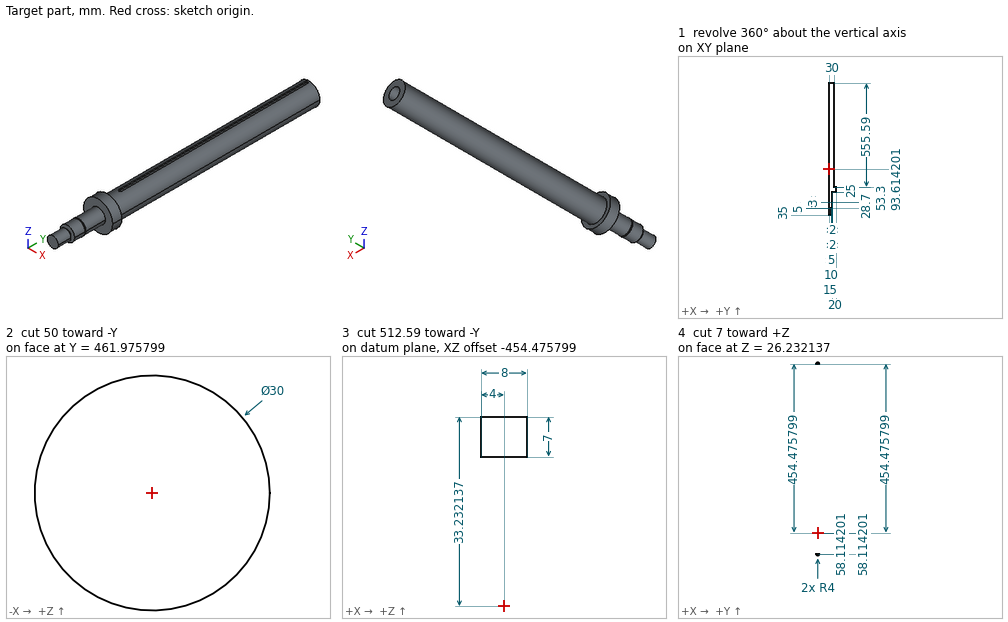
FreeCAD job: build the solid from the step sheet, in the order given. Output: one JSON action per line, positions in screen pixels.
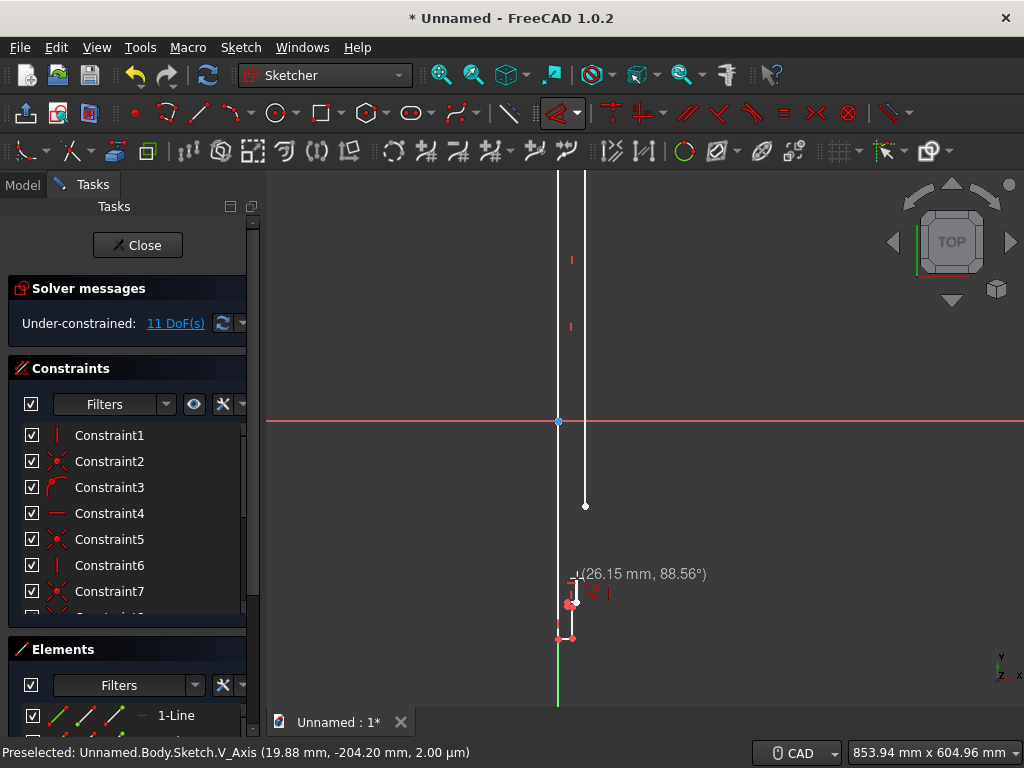
{"action": "left_click", "coordinate": [576, 577]}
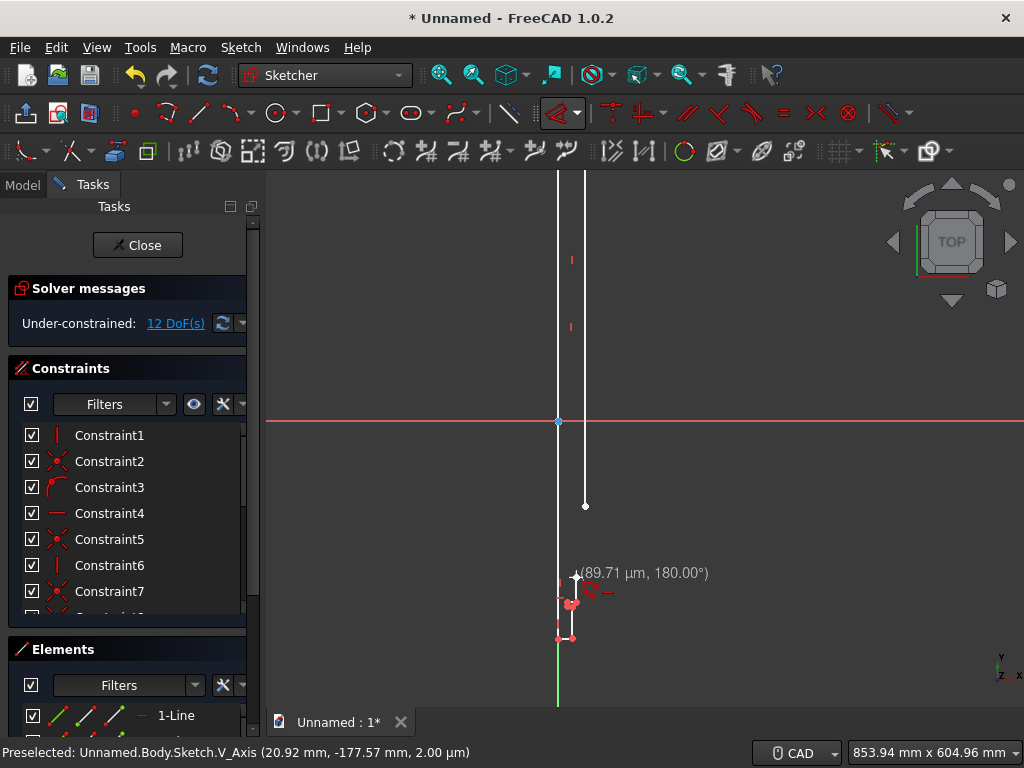
{"action": "scroll", "coordinate": [574, 577], "scroll_direction": "up", "scroll_amount": 11}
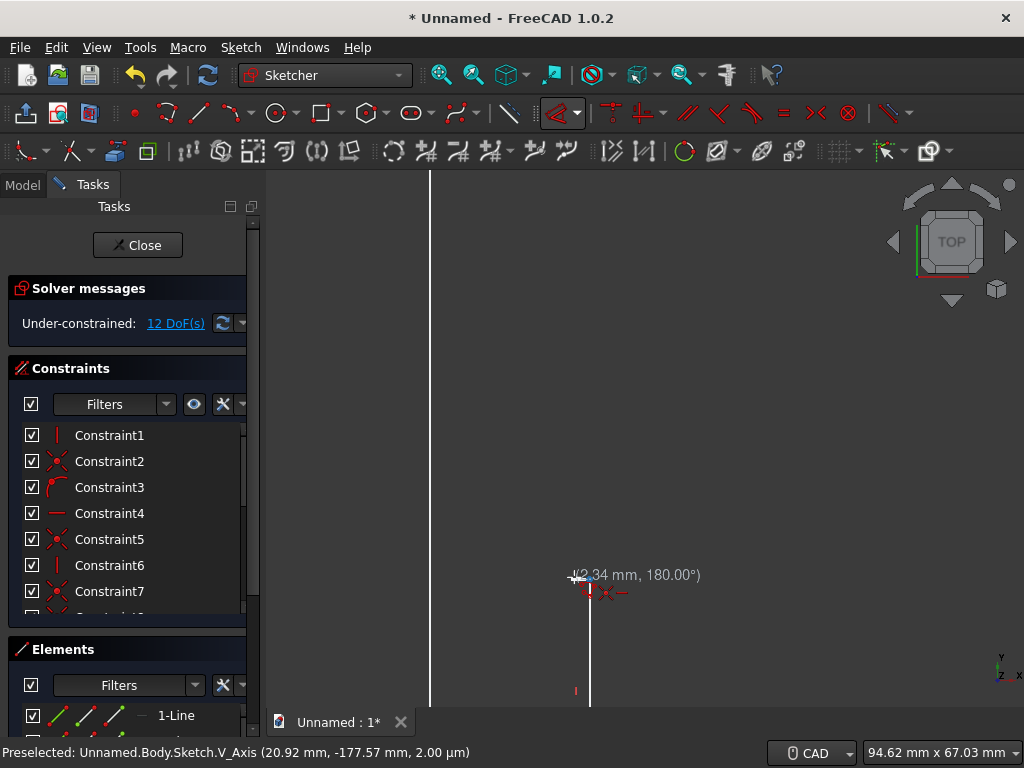
{"action": "left_click", "coordinate": [574, 571]}
{"action": "left_click", "coordinate": [574, 544]}
{"action": "left_click", "coordinate": [590, 544]}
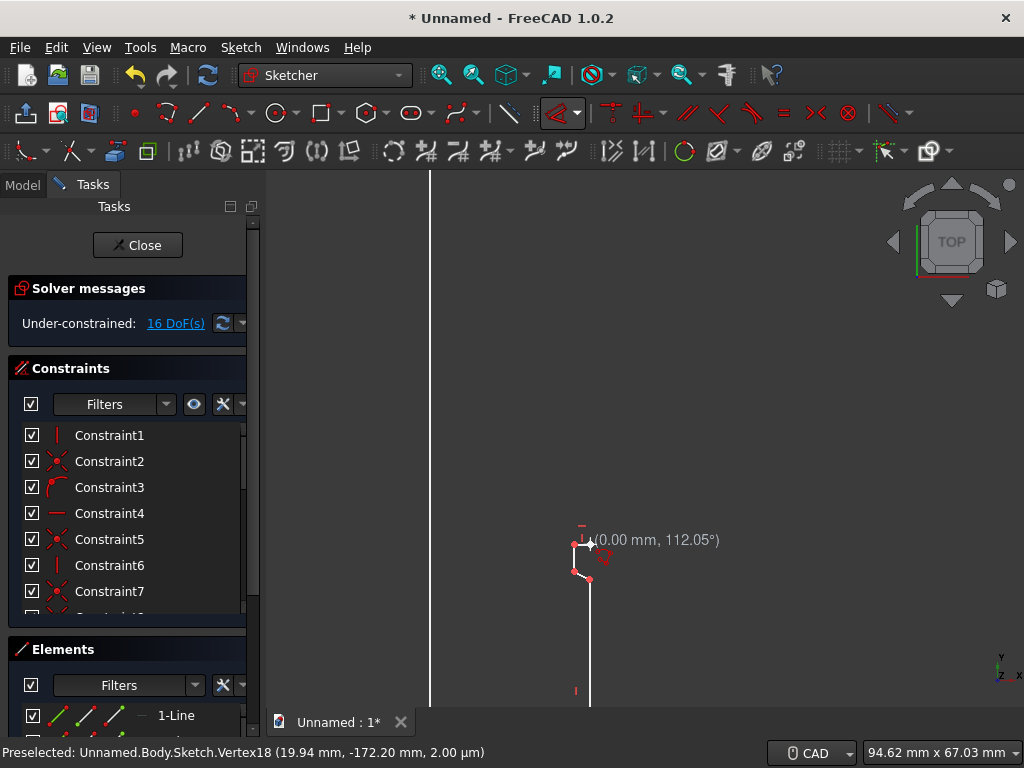
{"action": "scroll", "coordinate": [576, 577], "scroll_direction": "down", "scroll_amount": 14}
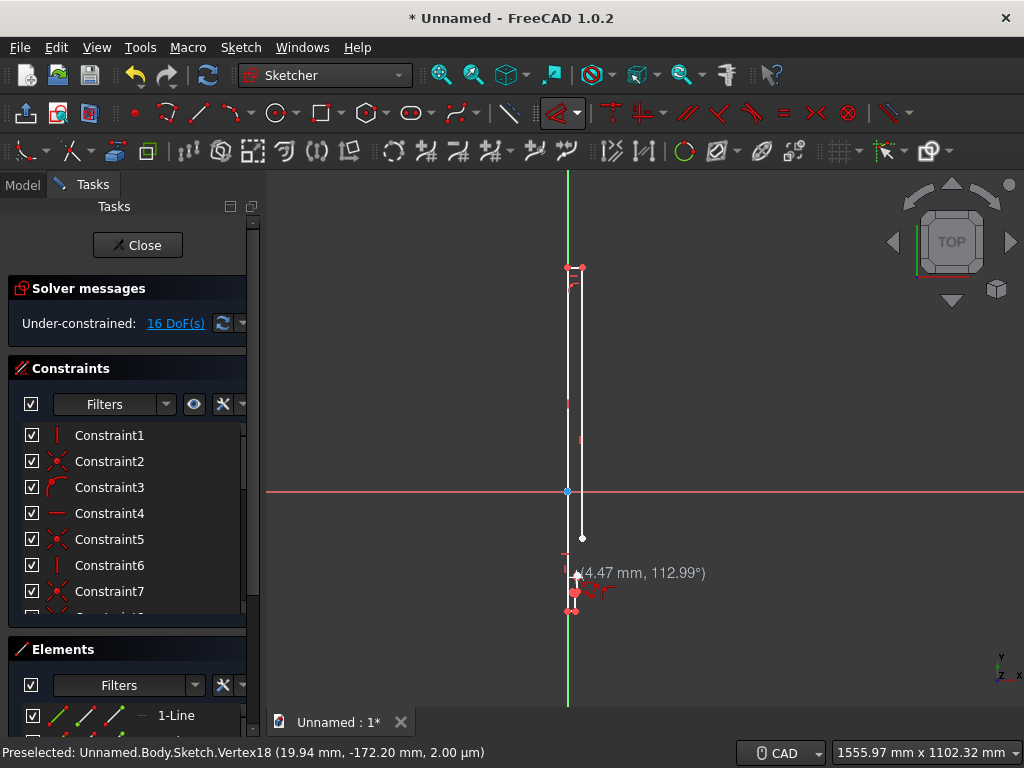
{"action": "scroll", "coordinate": [577, 550], "scroll_direction": "up", "scroll_amount": 3}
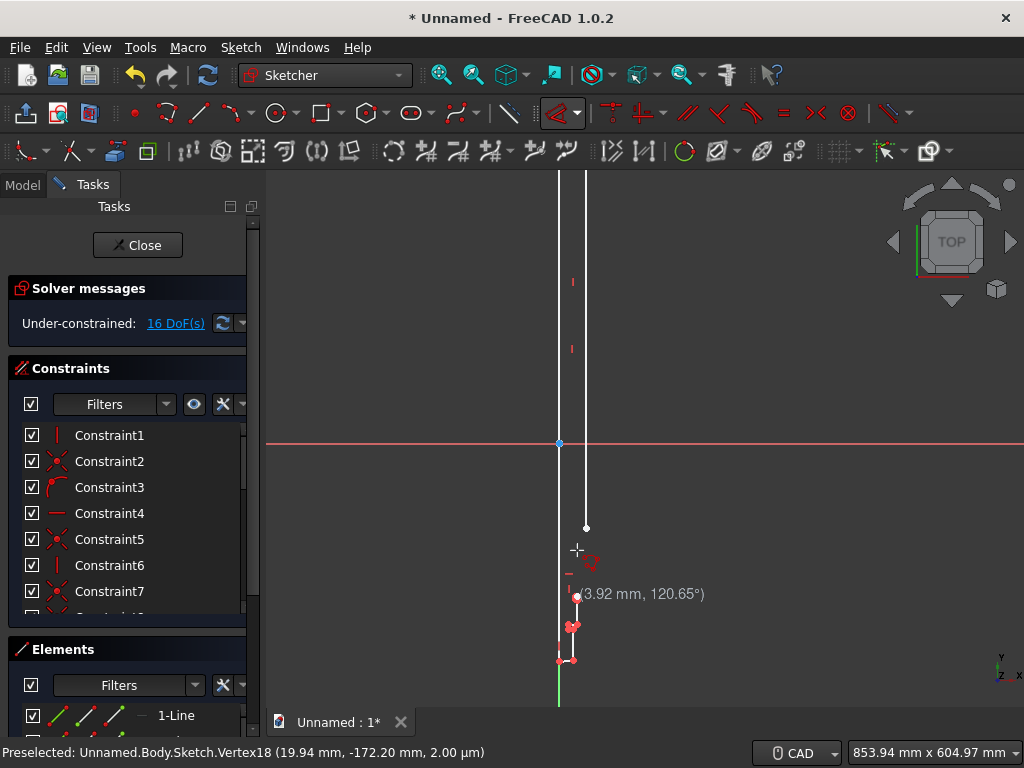
{"action": "left_click", "coordinate": [577, 549]}
{"action": "left_click", "coordinate": [595, 549]}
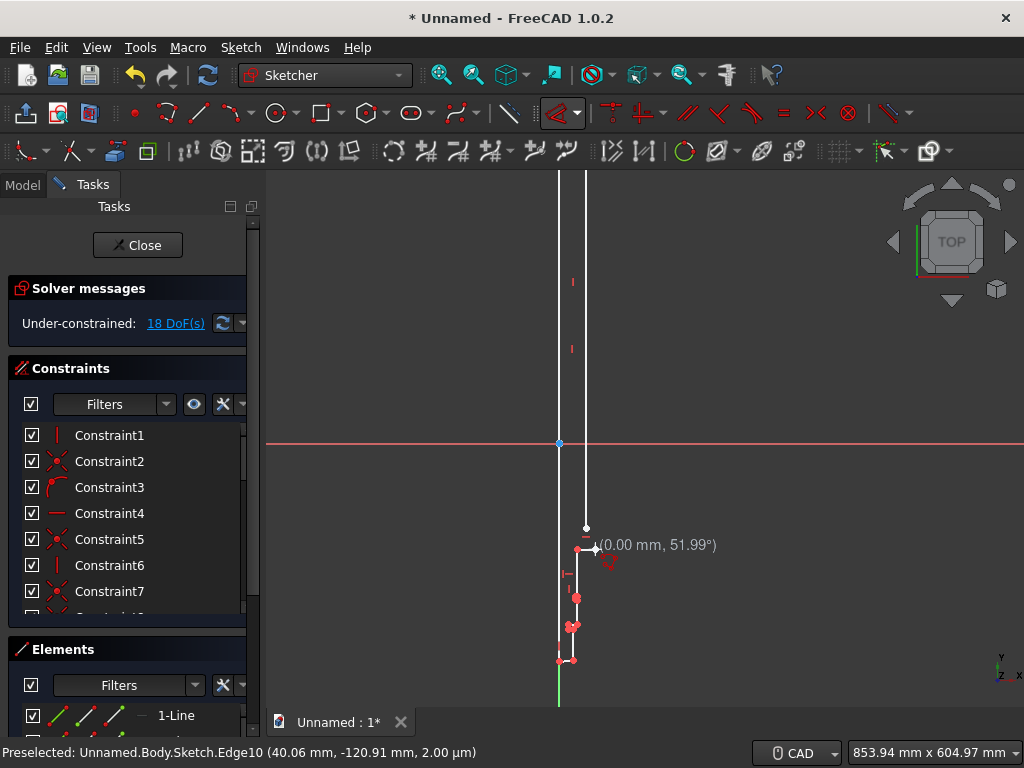
{"action": "scroll", "coordinate": [595, 527], "scroll_direction": "up", "scroll_amount": 3}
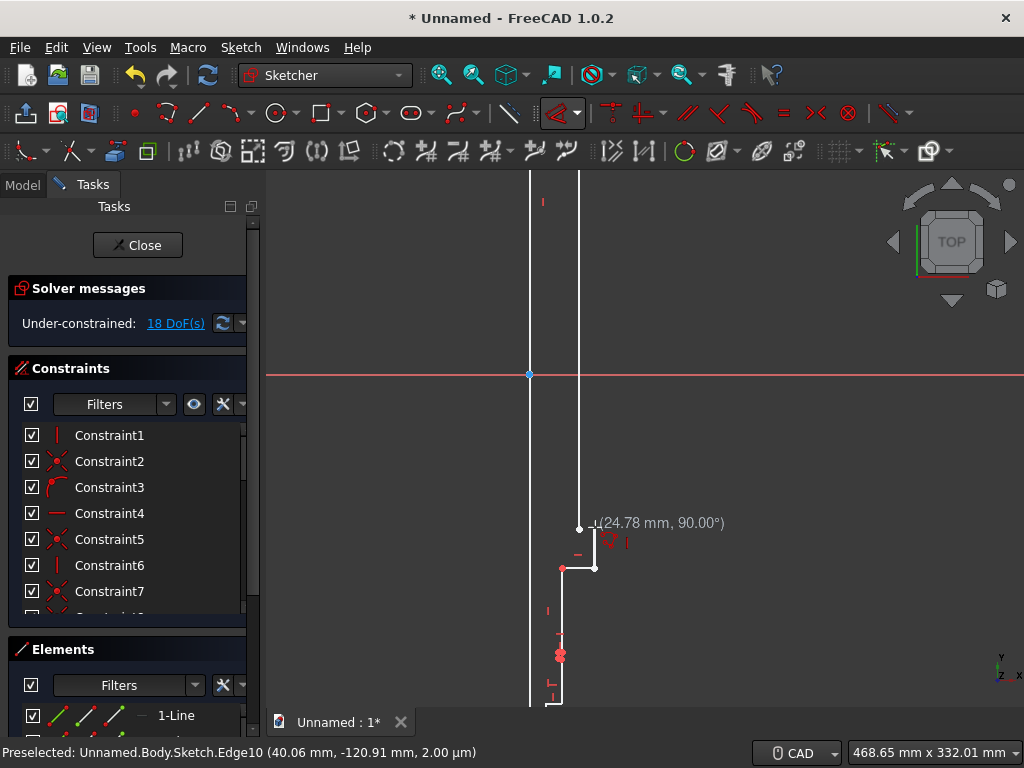
{"action": "left_click", "coordinate": [595, 526]}
{"action": "left_click", "coordinate": [579, 530]}
{"action": "key", "text": "Escape"}
{"action": "key", "text": "Escape"}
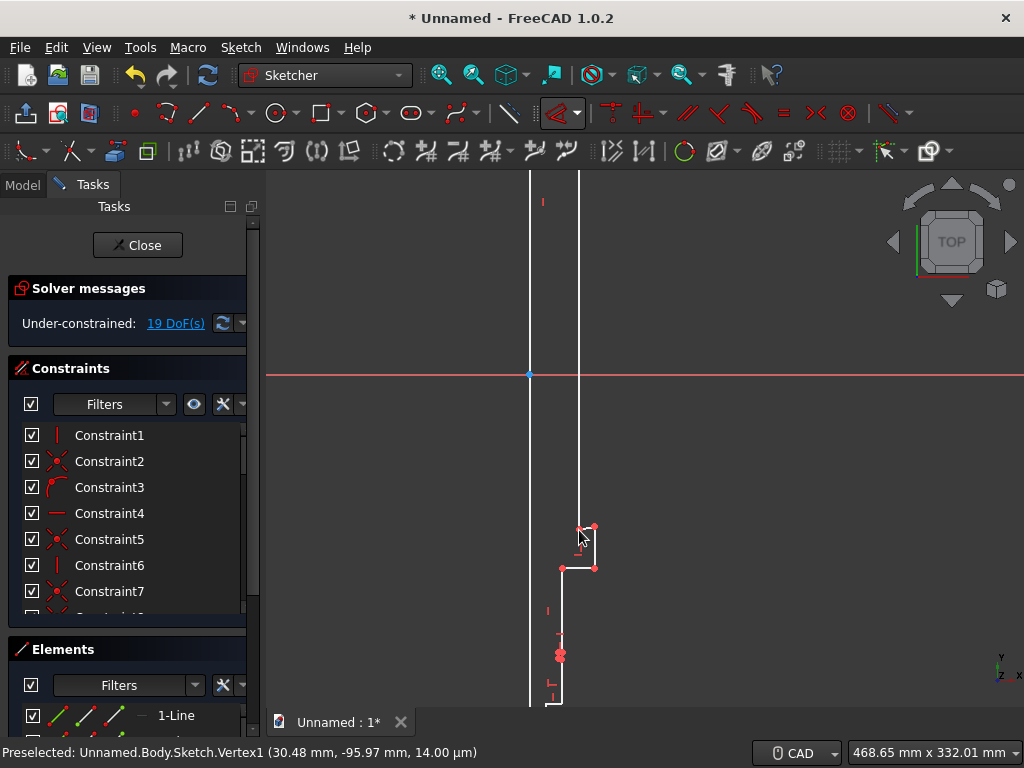
{"action": "scroll", "coordinate": [583, 542], "scroll_direction": "down", "scroll_amount": 6}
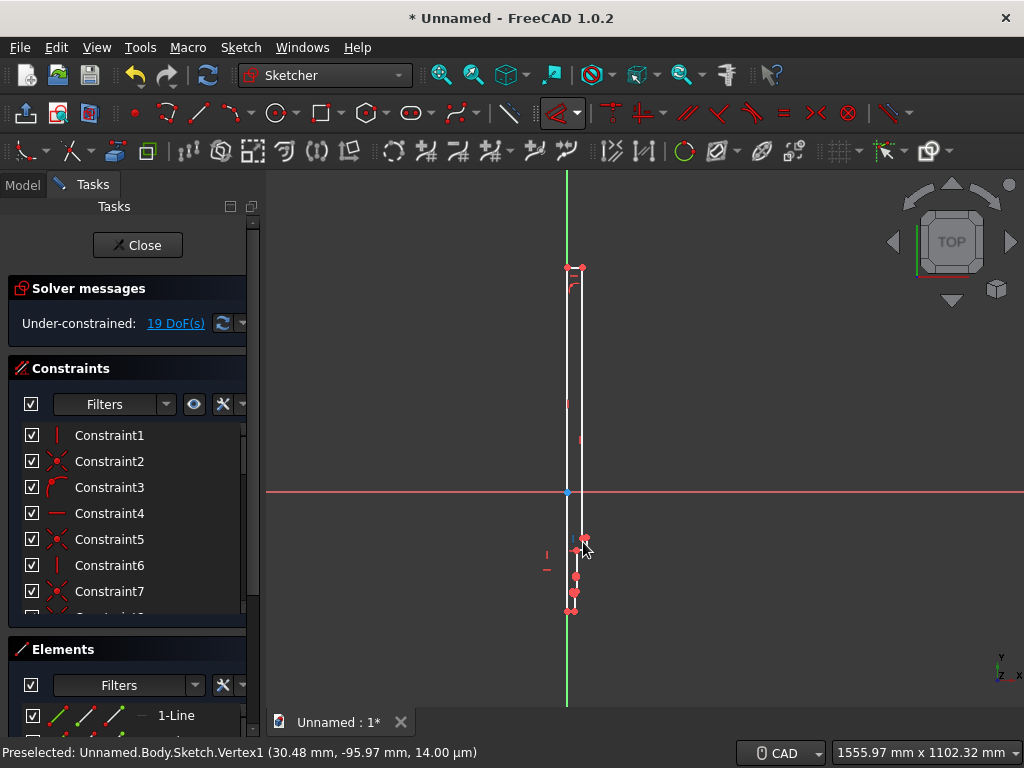
{"action": "scroll", "coordinate": [570, 612], "scroll_direction": "up", "scroll_amount": 8}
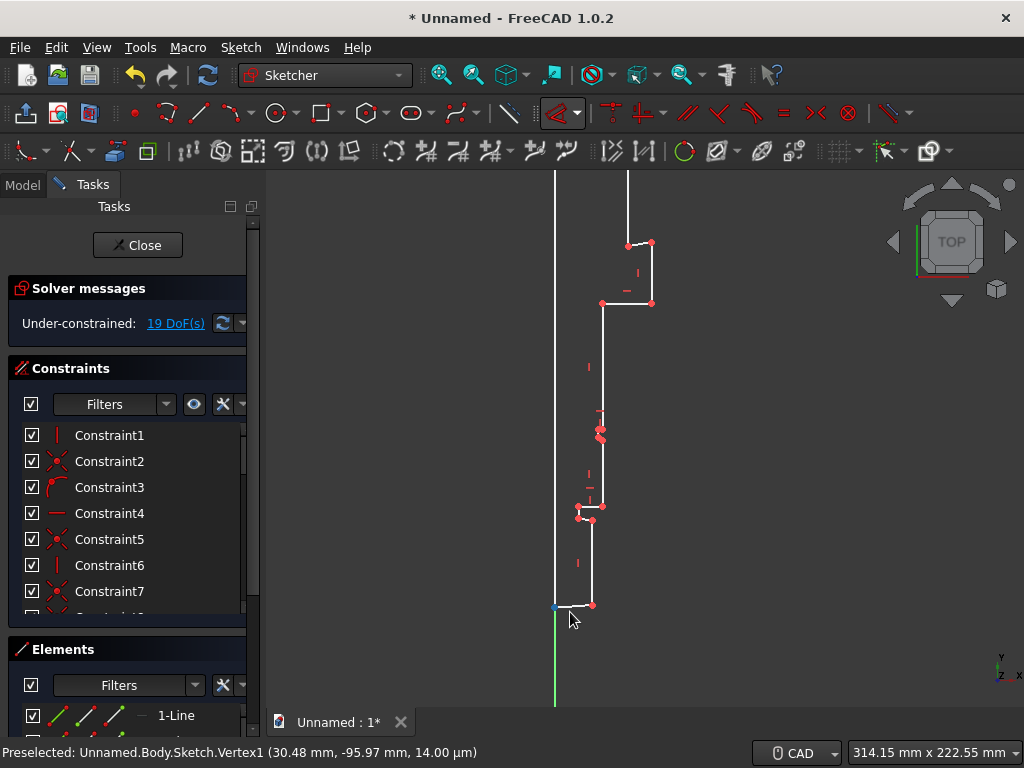
{"action": "left_click", "coordinate": [570, 607]}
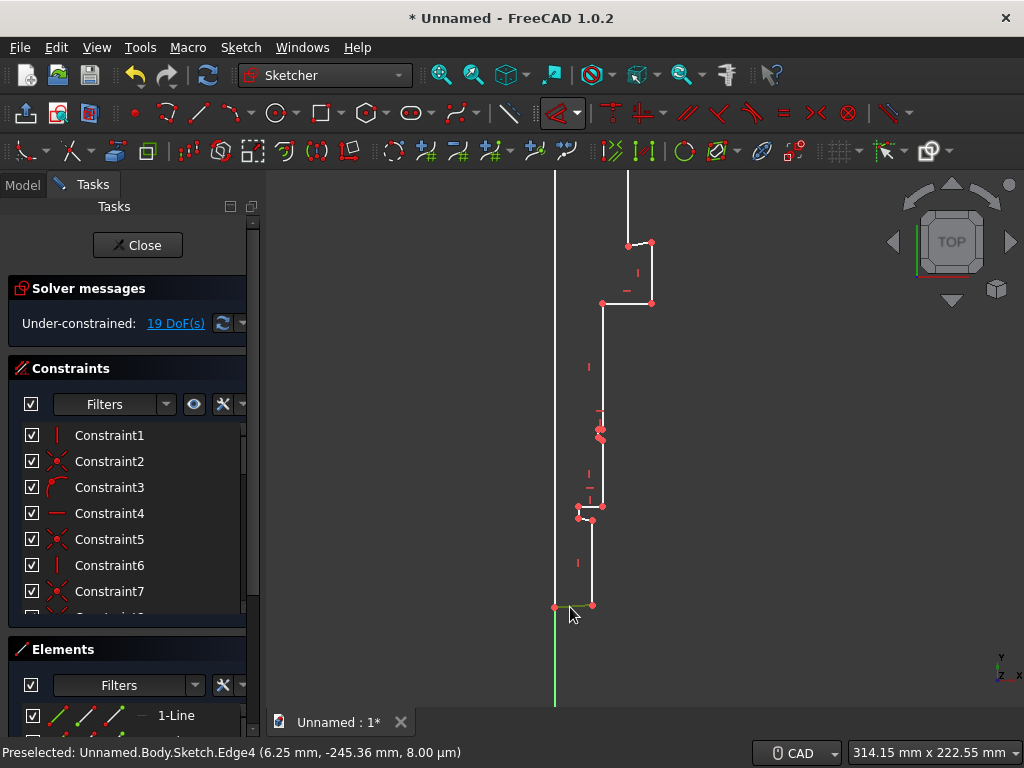
{"action": "left_click", "coordinate": [666, 114]}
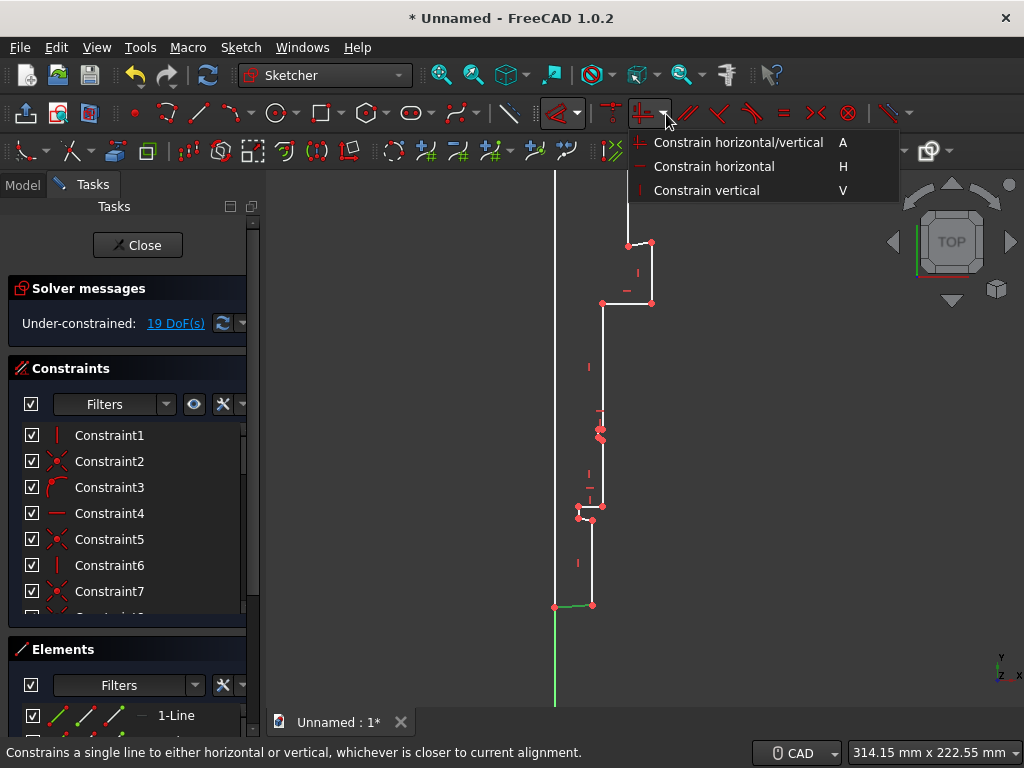
{"action": "left_click", "coordinate": [764, 166]}